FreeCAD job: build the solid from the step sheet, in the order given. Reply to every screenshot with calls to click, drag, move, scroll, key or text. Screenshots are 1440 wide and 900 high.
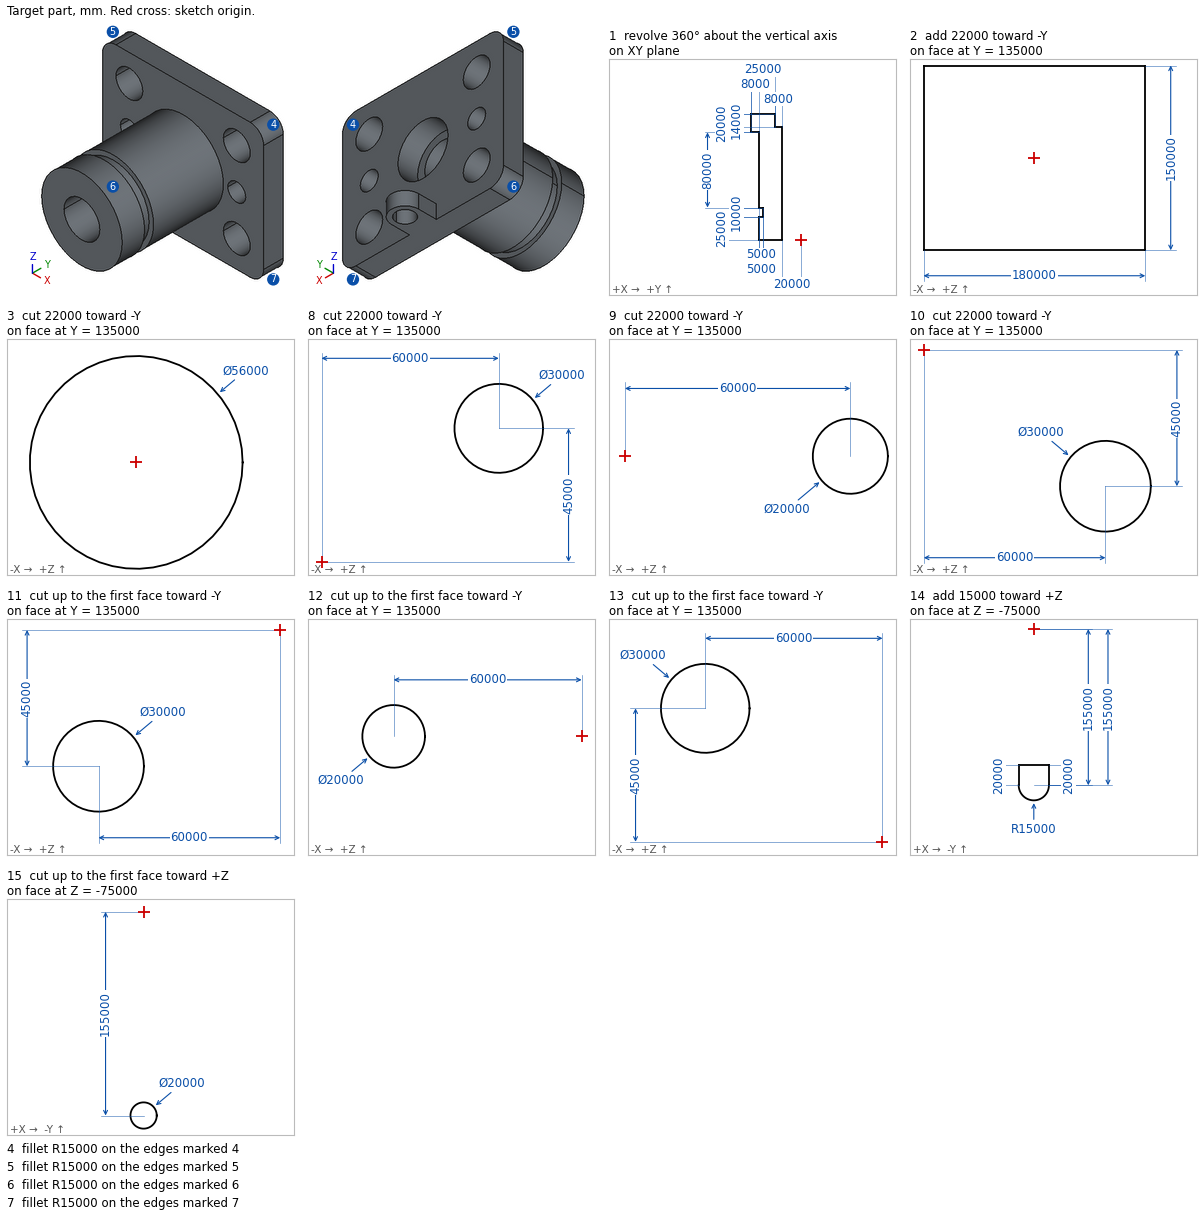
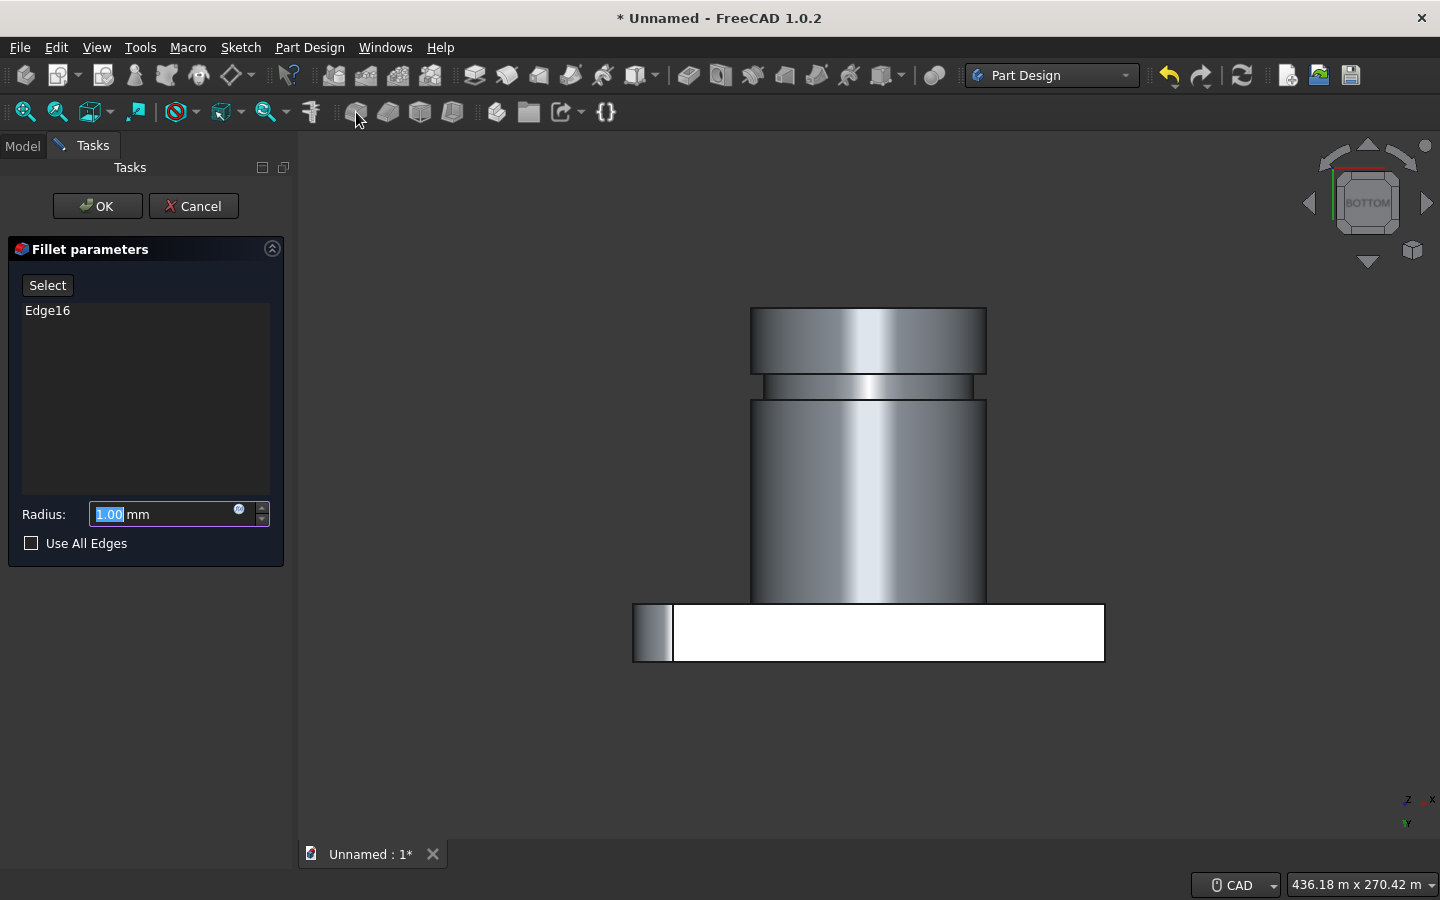
text(15000)
key(Tab)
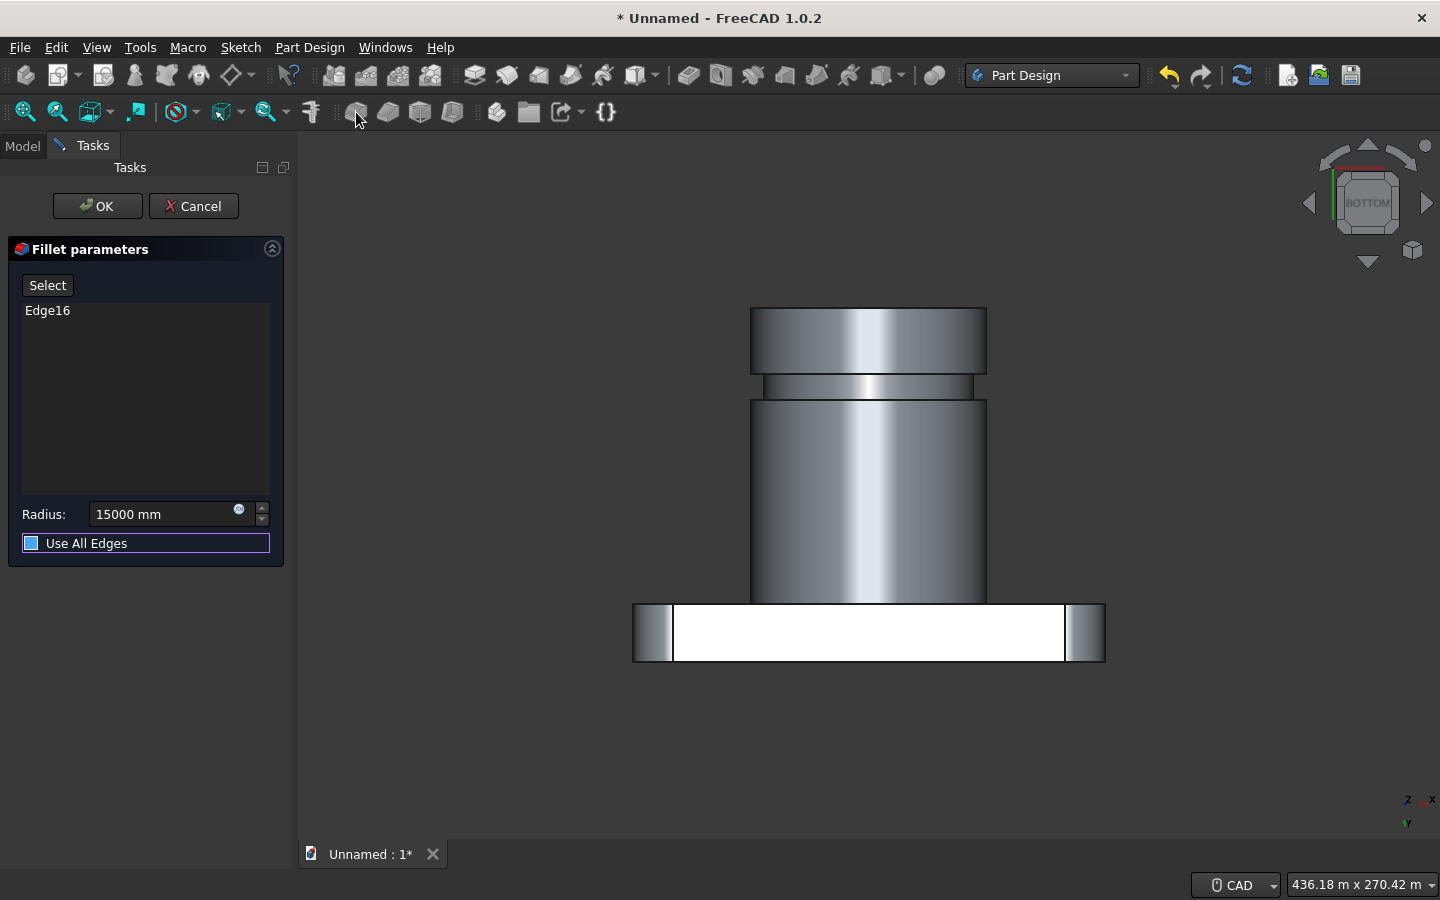
click(98, 206)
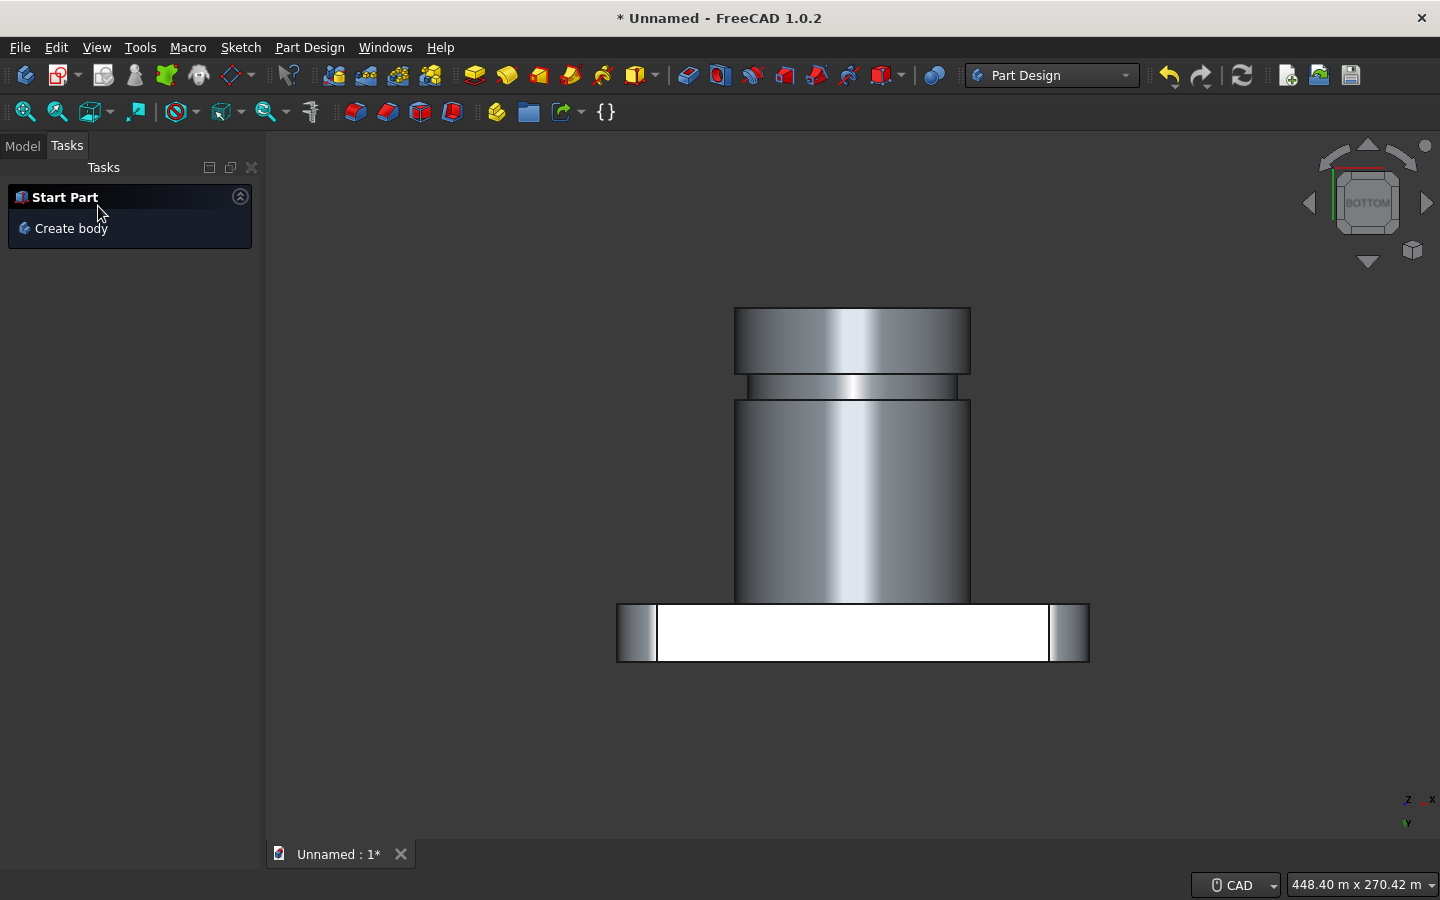
key(4)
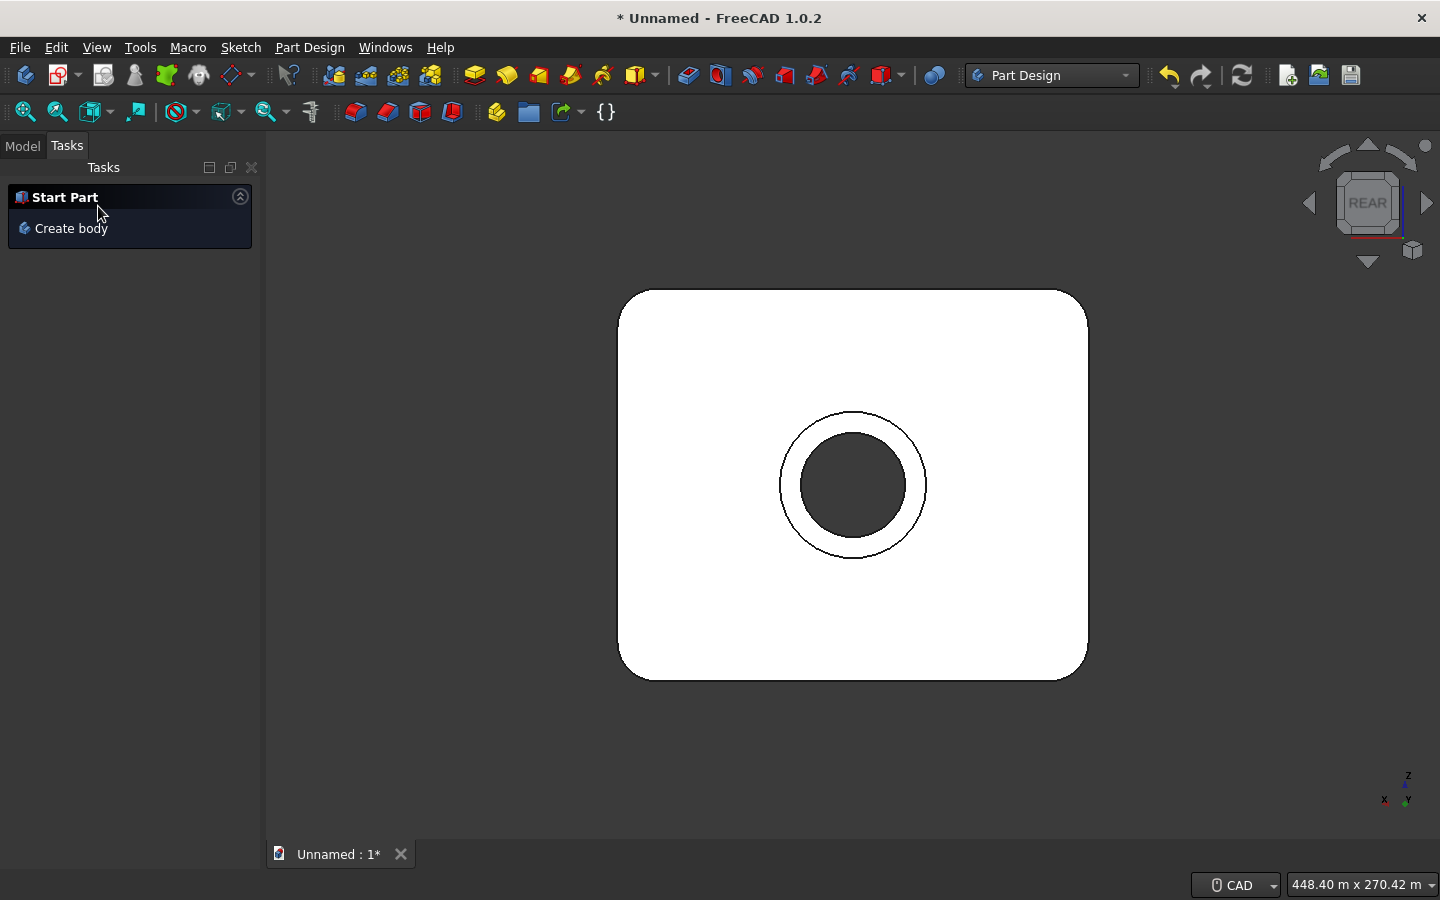
click(718, 372)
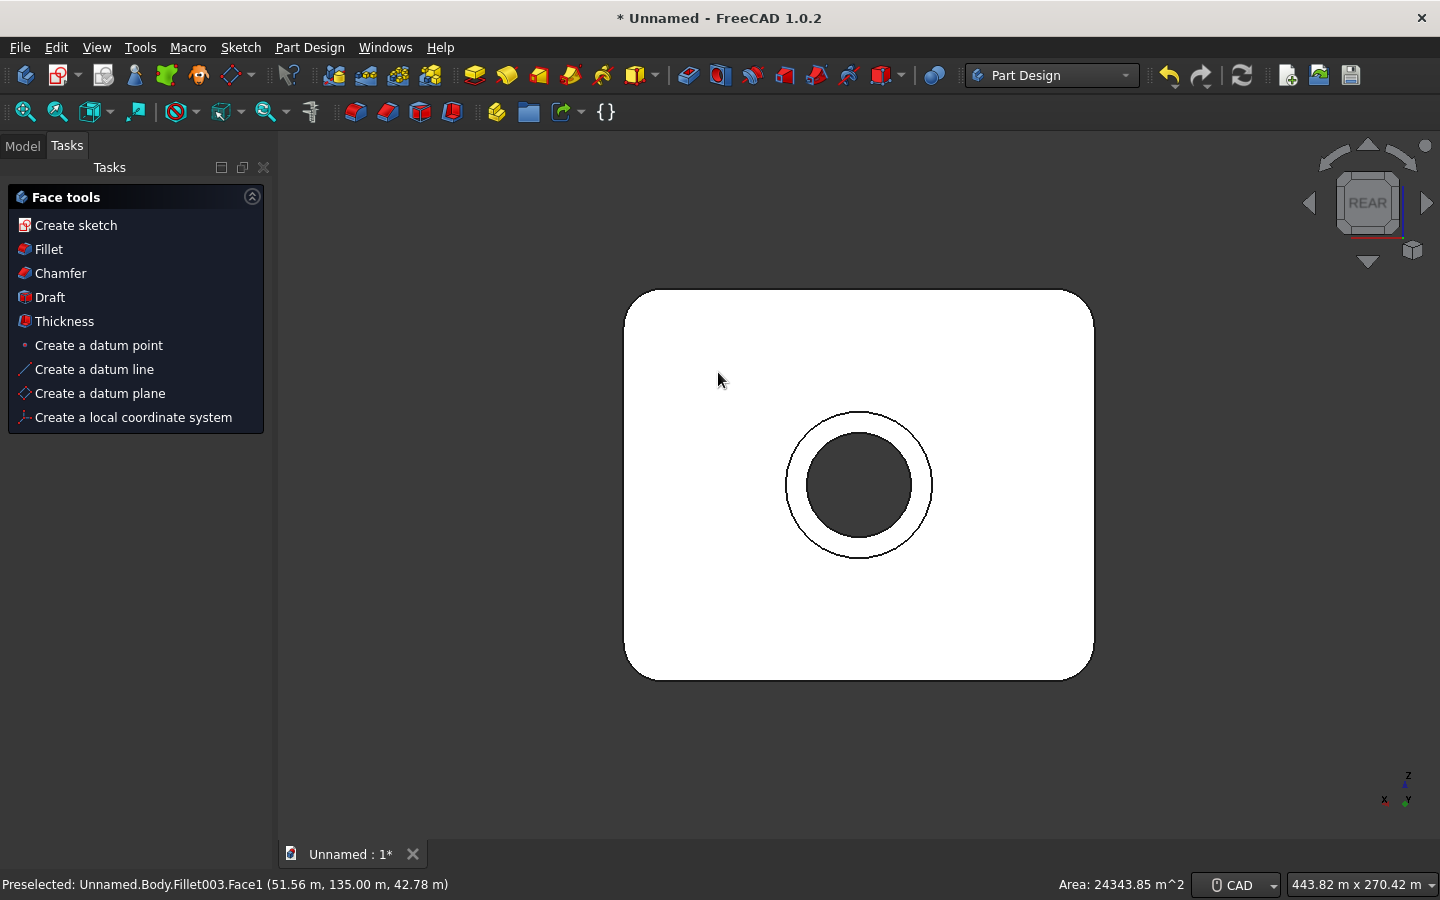
click(58, 76)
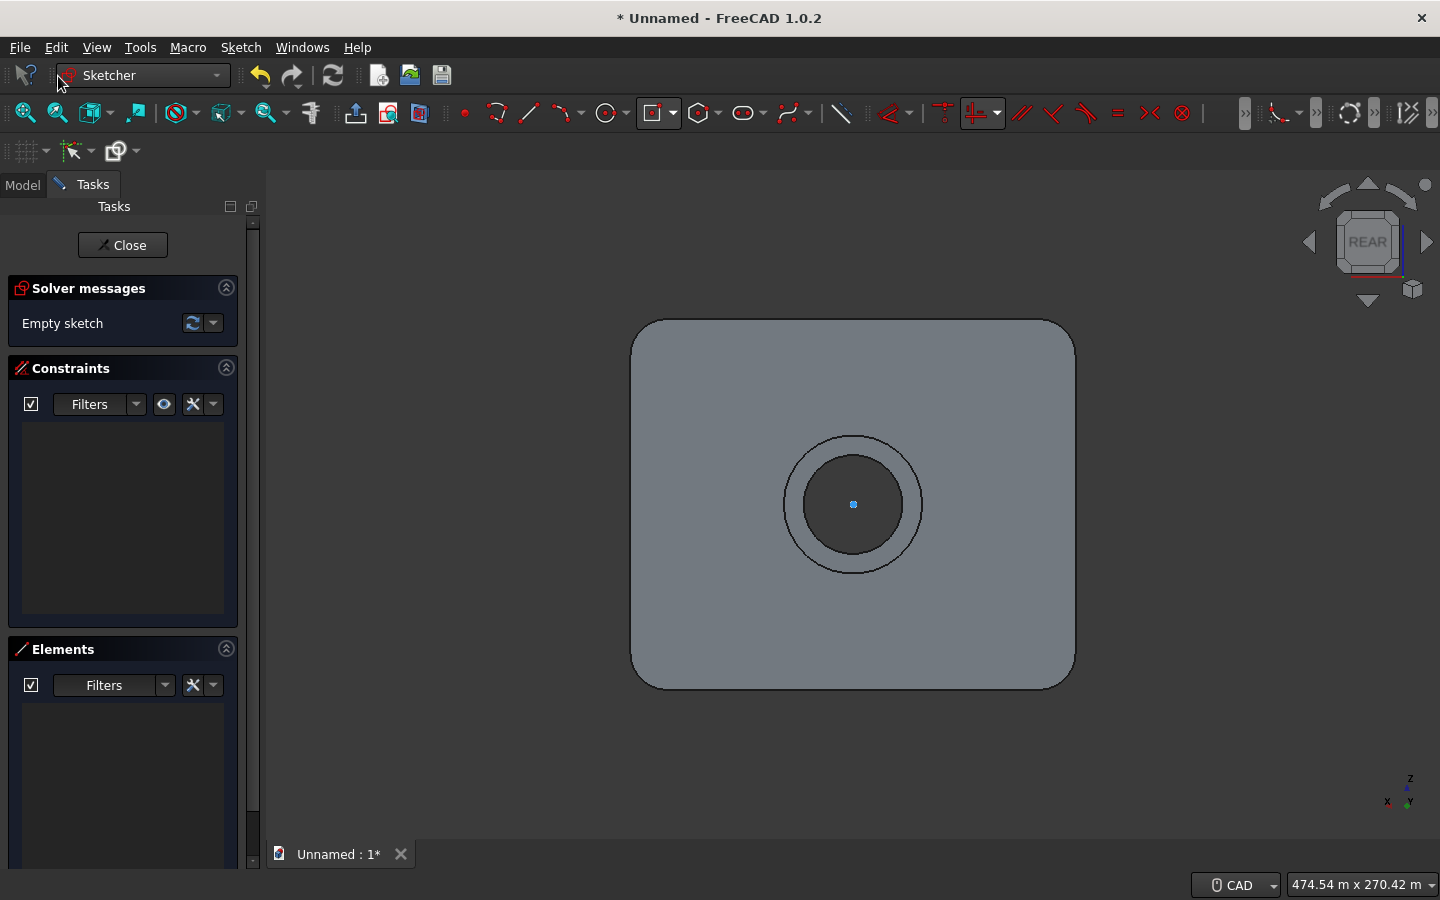
scroll(1044, 371, up, 9)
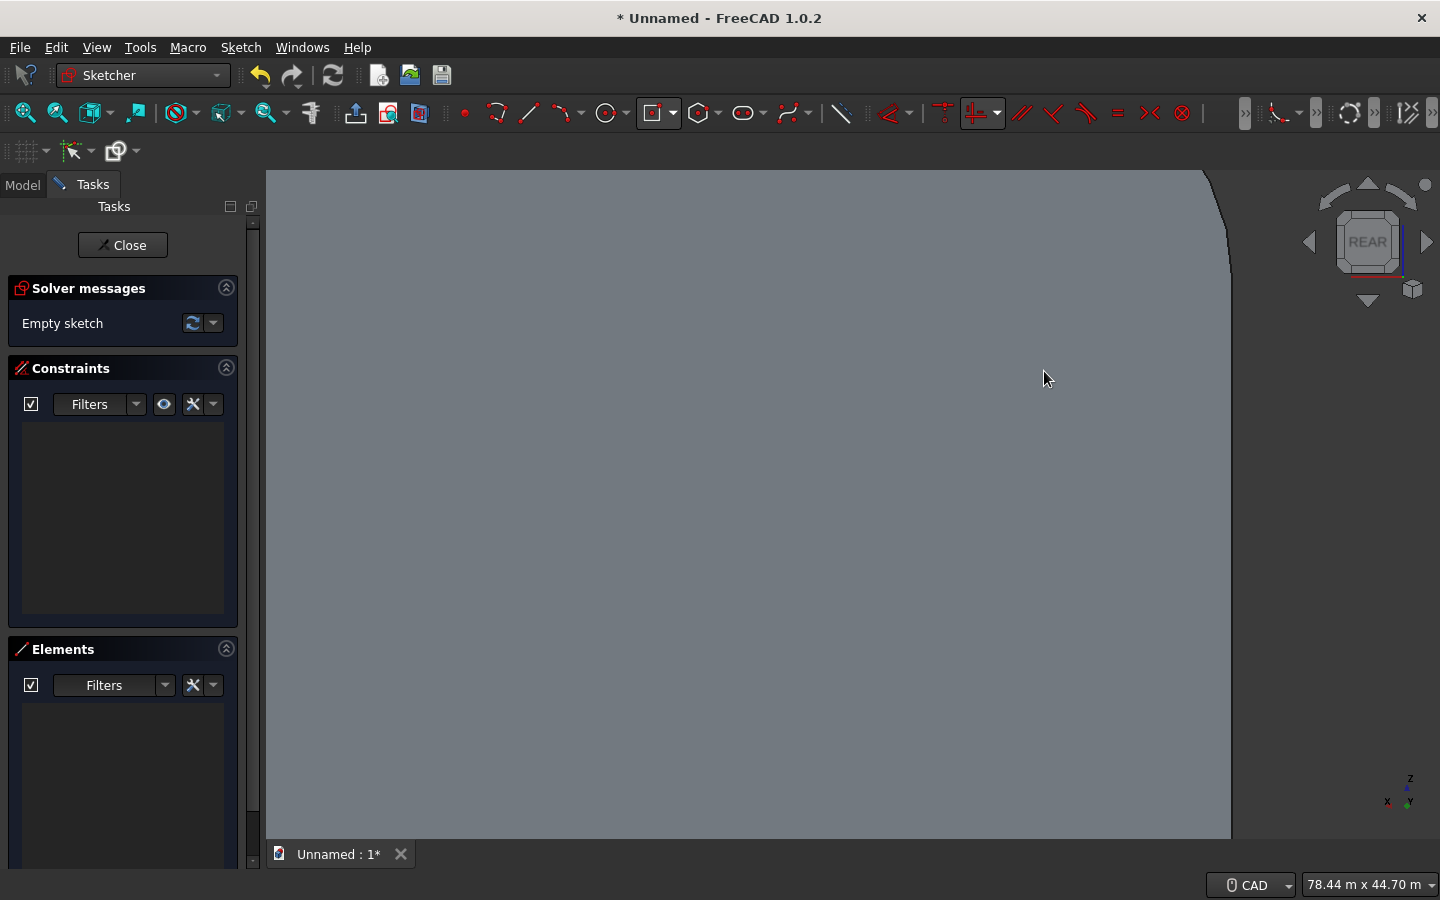
click(606, 114)